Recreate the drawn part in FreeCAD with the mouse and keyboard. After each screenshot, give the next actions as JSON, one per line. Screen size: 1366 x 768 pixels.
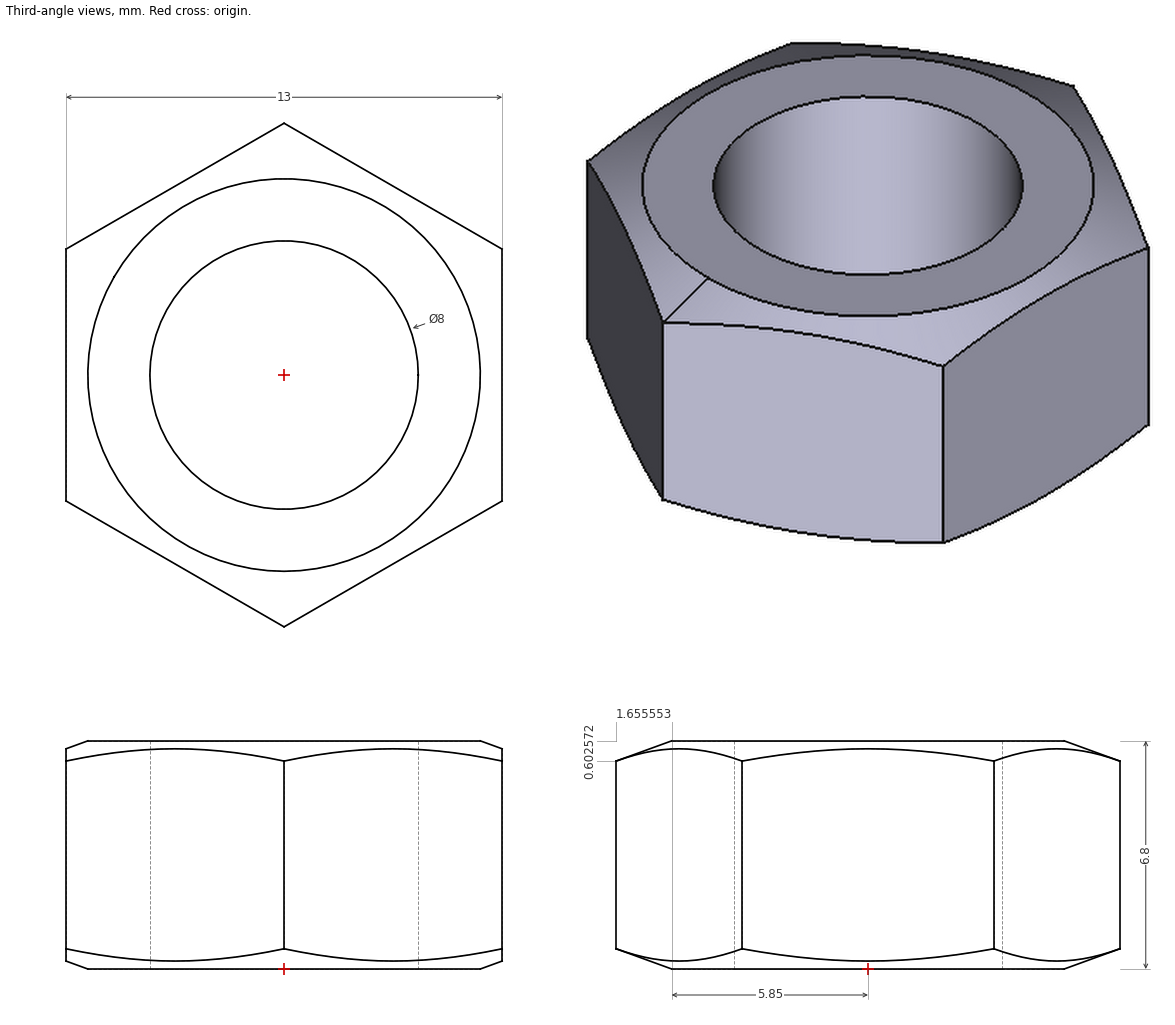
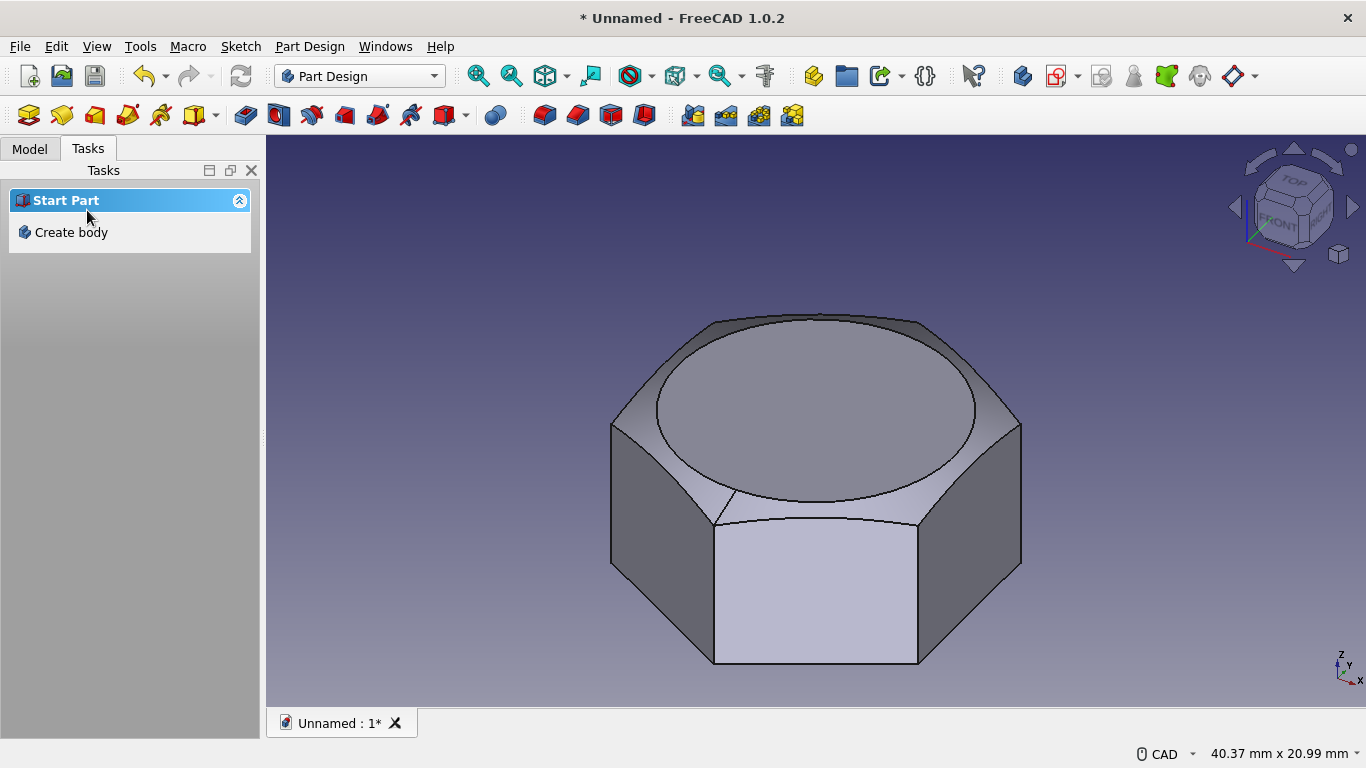
{"action": "key", "text": "v f"}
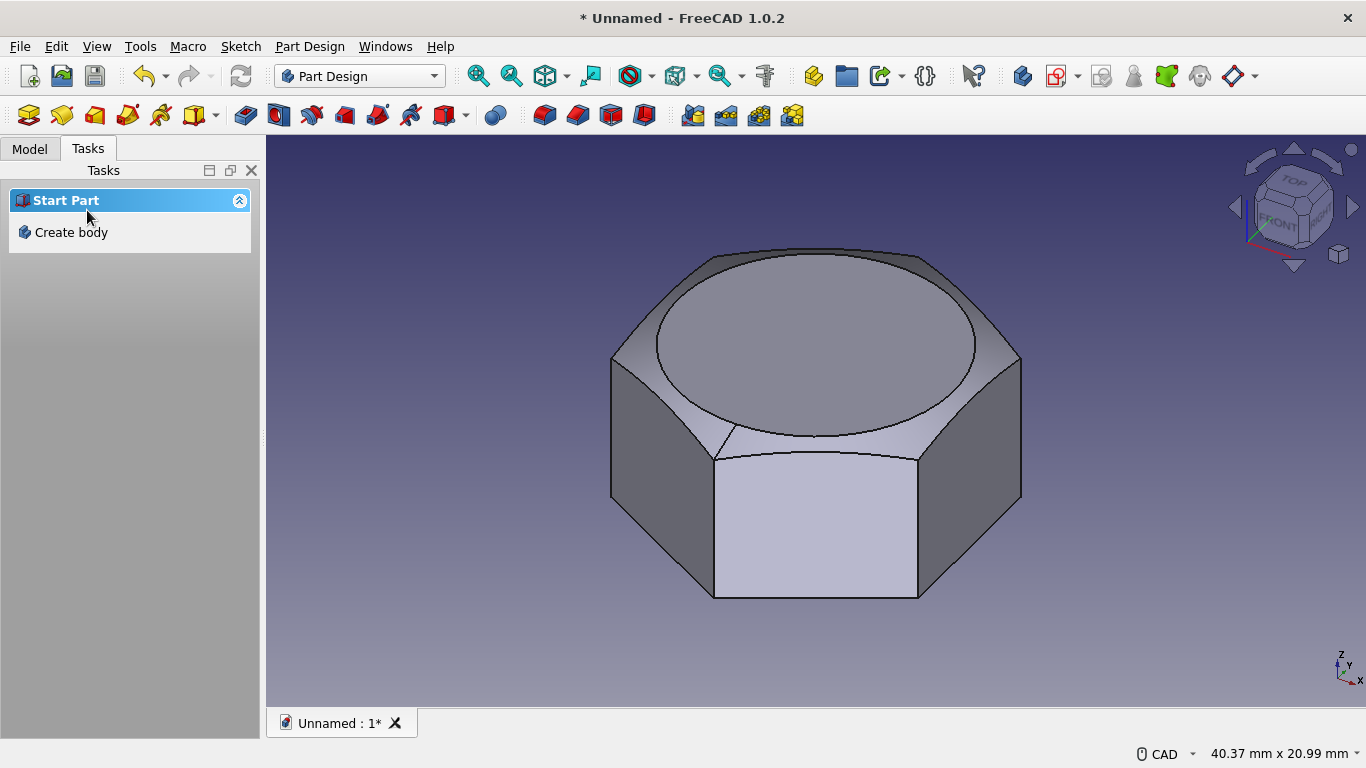
{"action": "left_click", "coordinate": [30, 148]}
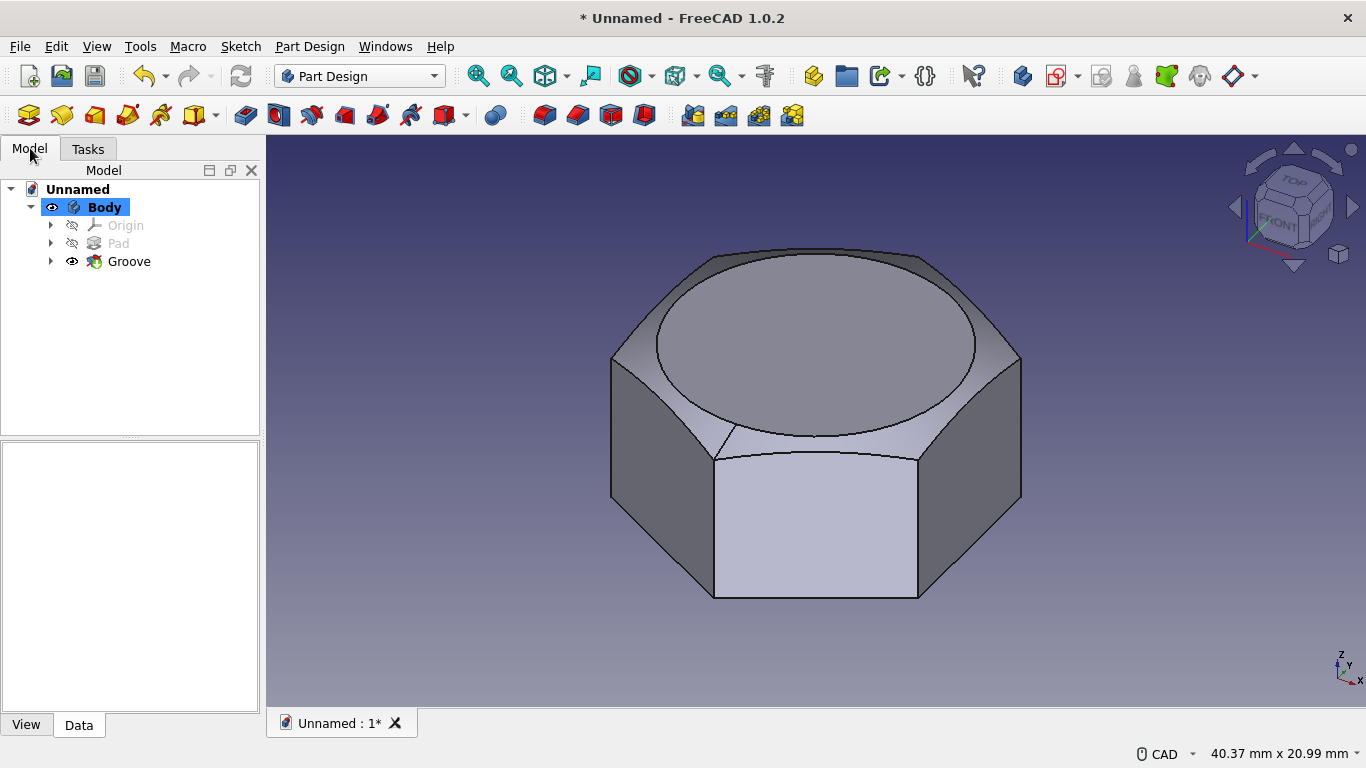
{"action": "left_click", "coordinate": [51, 225]}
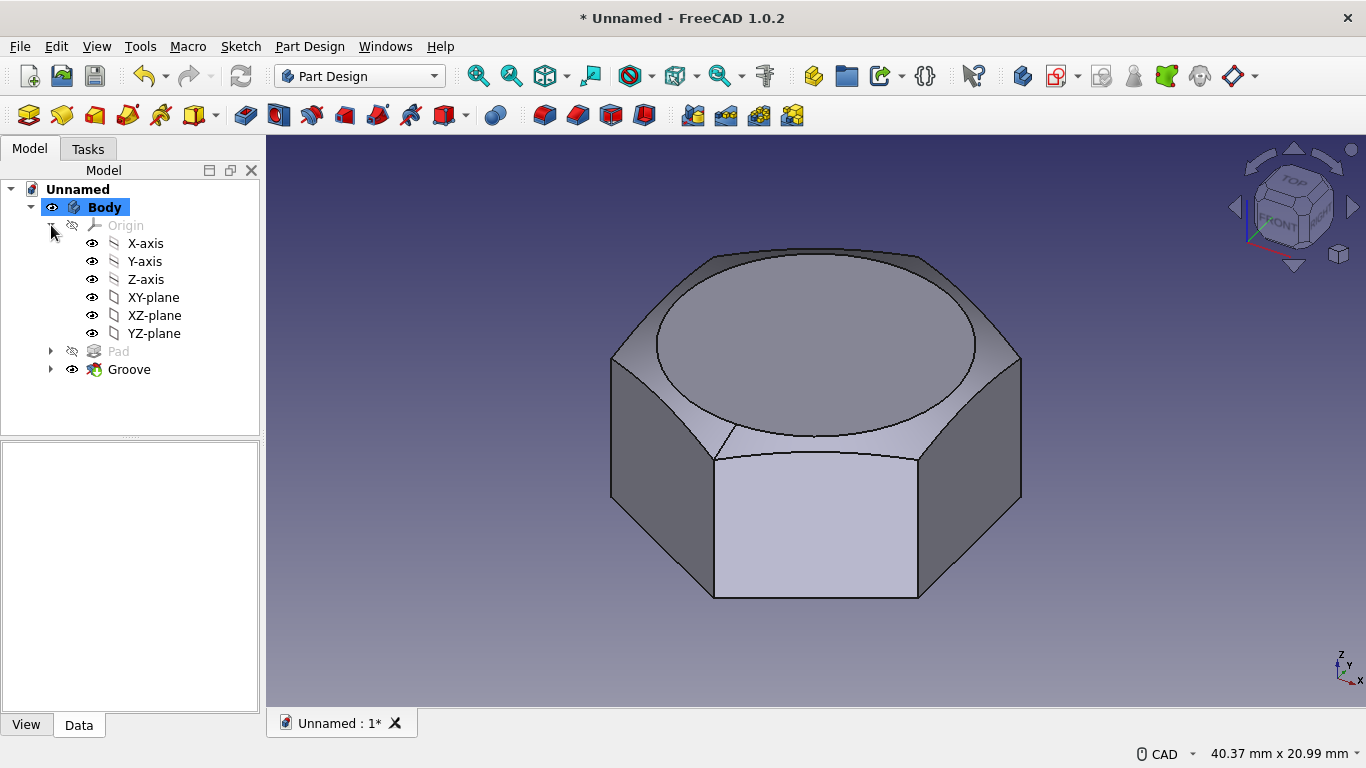
{"action": "left_click", "coordinate": [137, 297]}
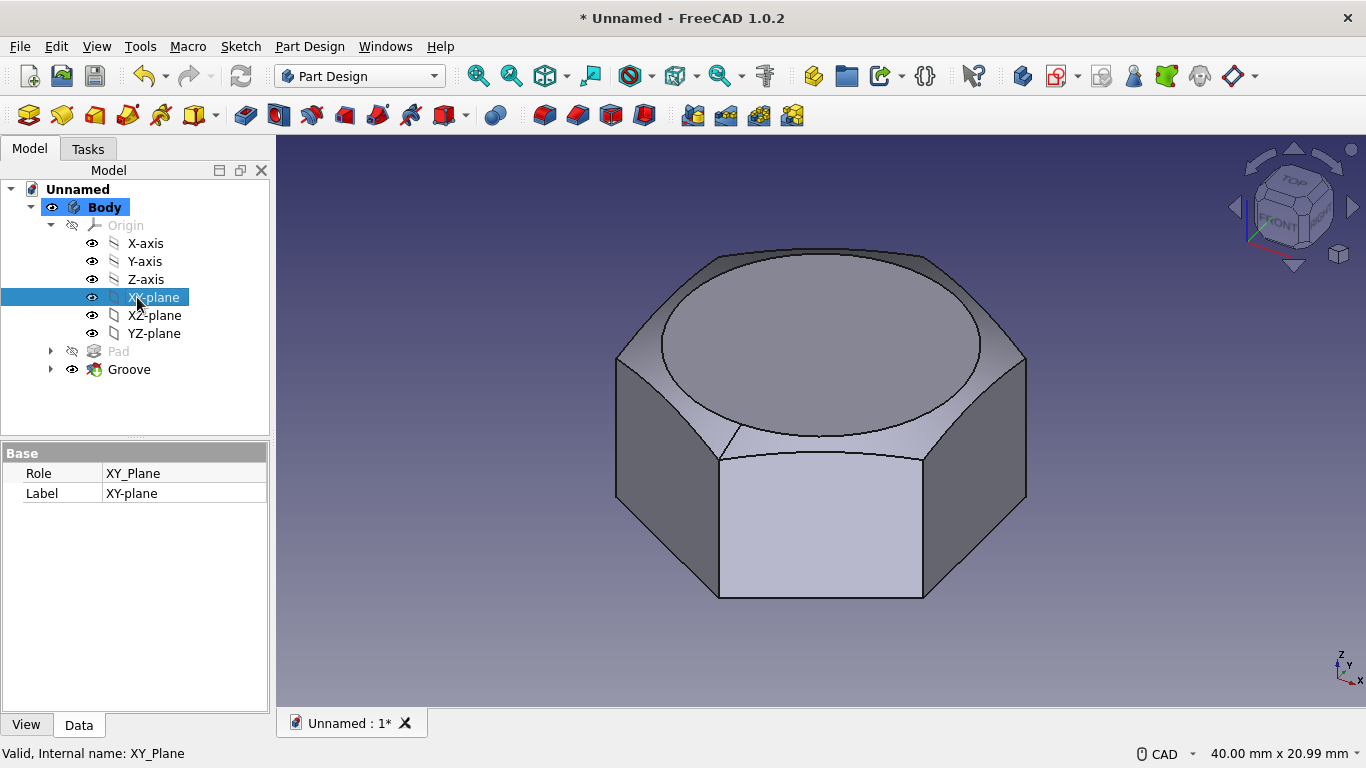
{"action": "left_click", "coordinate": [1232, 76]}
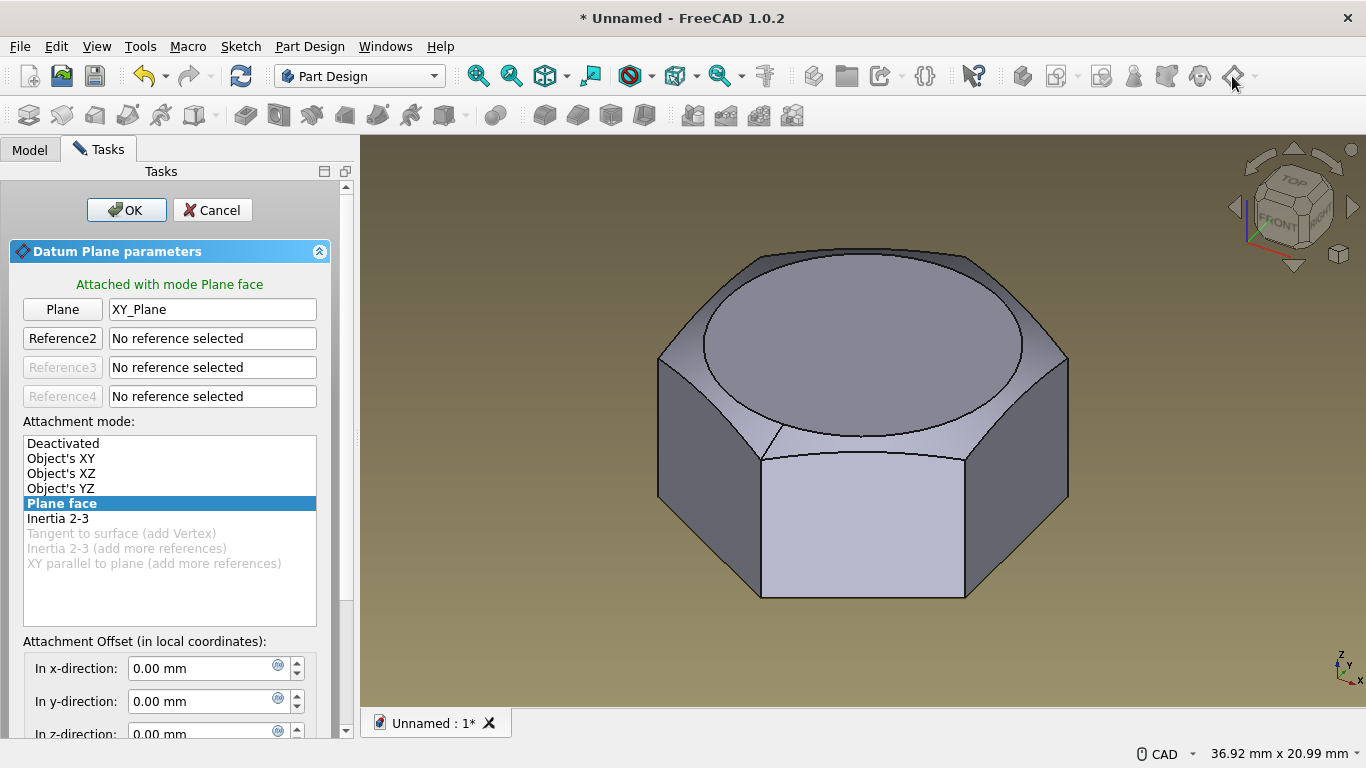
{"action": "scroll", "coordinate": [346, 460], "scroll_direction": "down", "scroll_amount": 2}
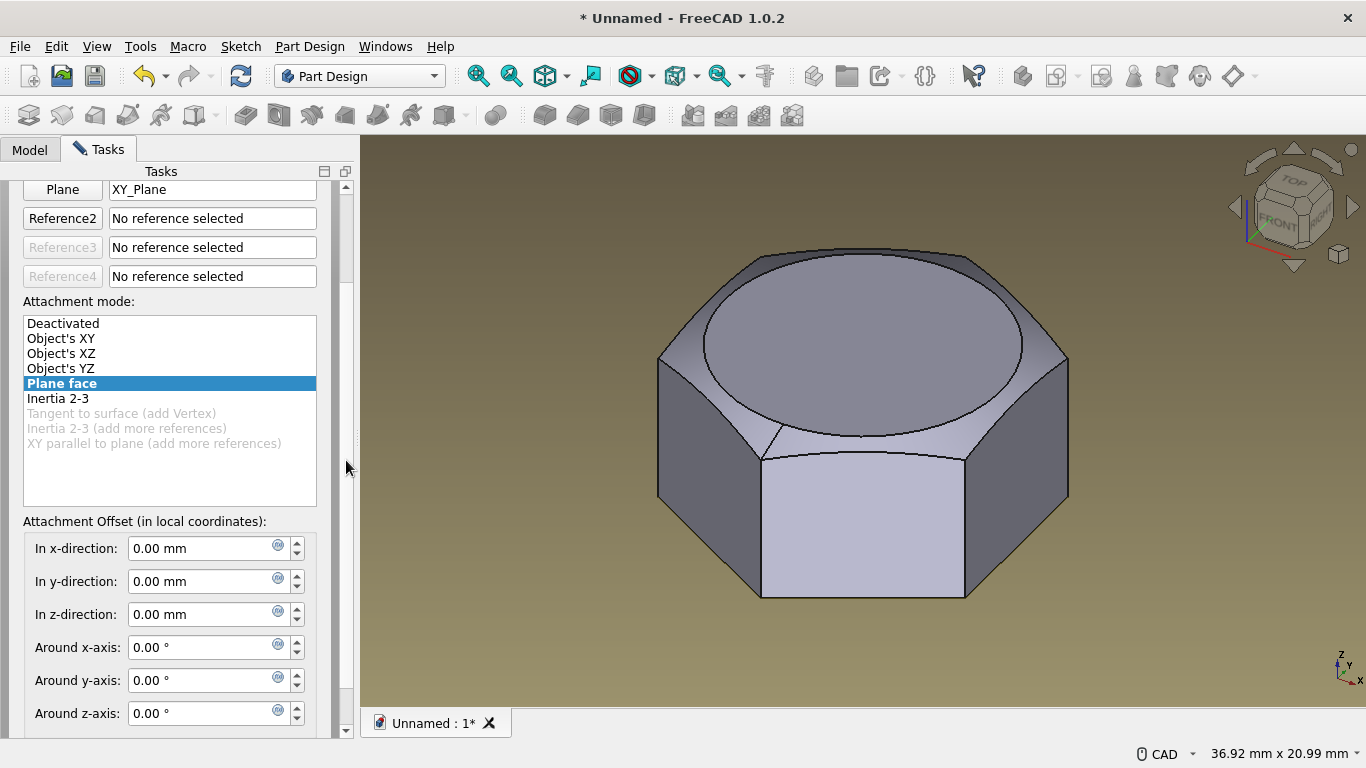
{"action": "triple_click", "coordinate": [210, 614]}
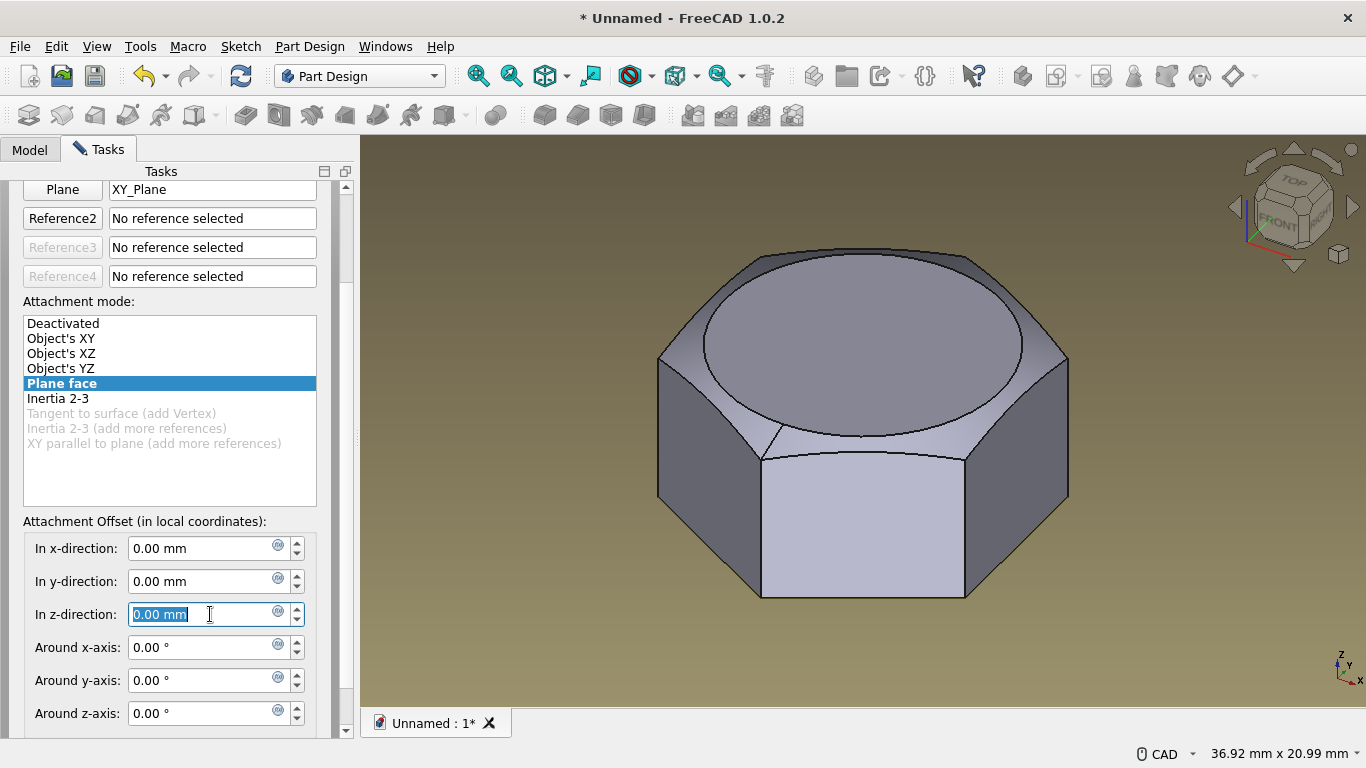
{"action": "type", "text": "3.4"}
{"action": "key", "text": "Tab"}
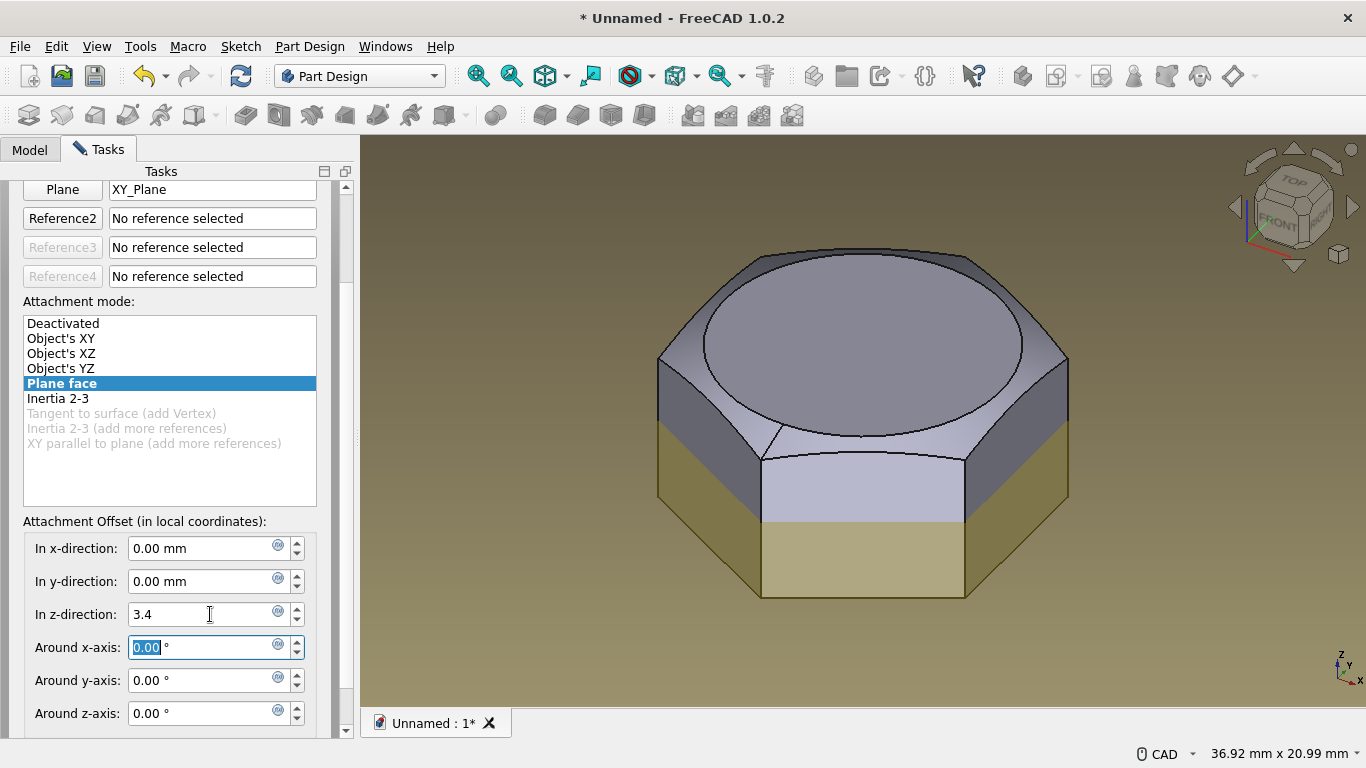
{"action": "scroll", "coordinate": [346, 460], "scroll_direction": "up", "scroll_amount": 3}